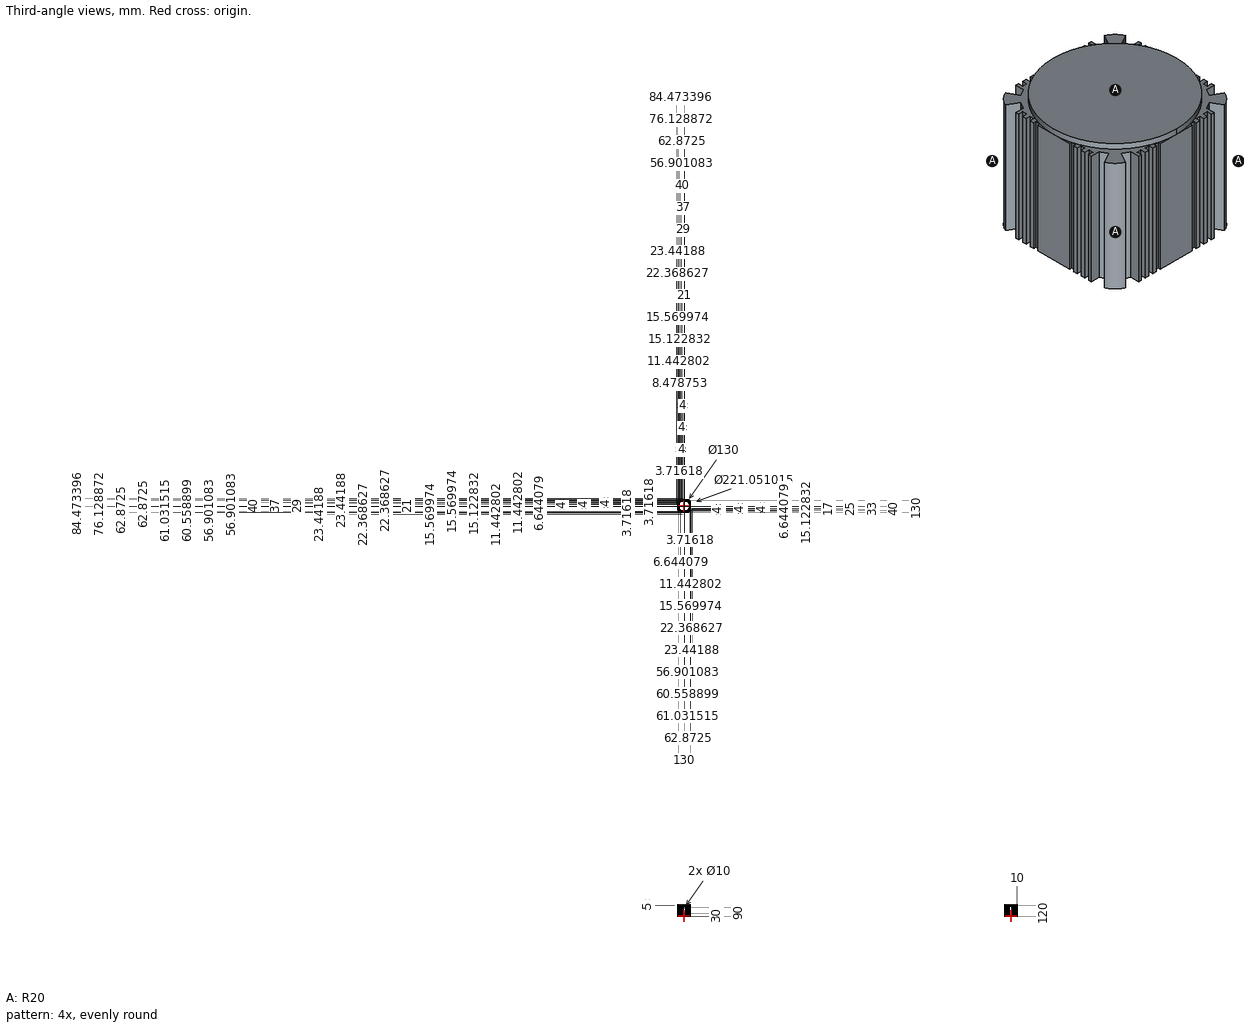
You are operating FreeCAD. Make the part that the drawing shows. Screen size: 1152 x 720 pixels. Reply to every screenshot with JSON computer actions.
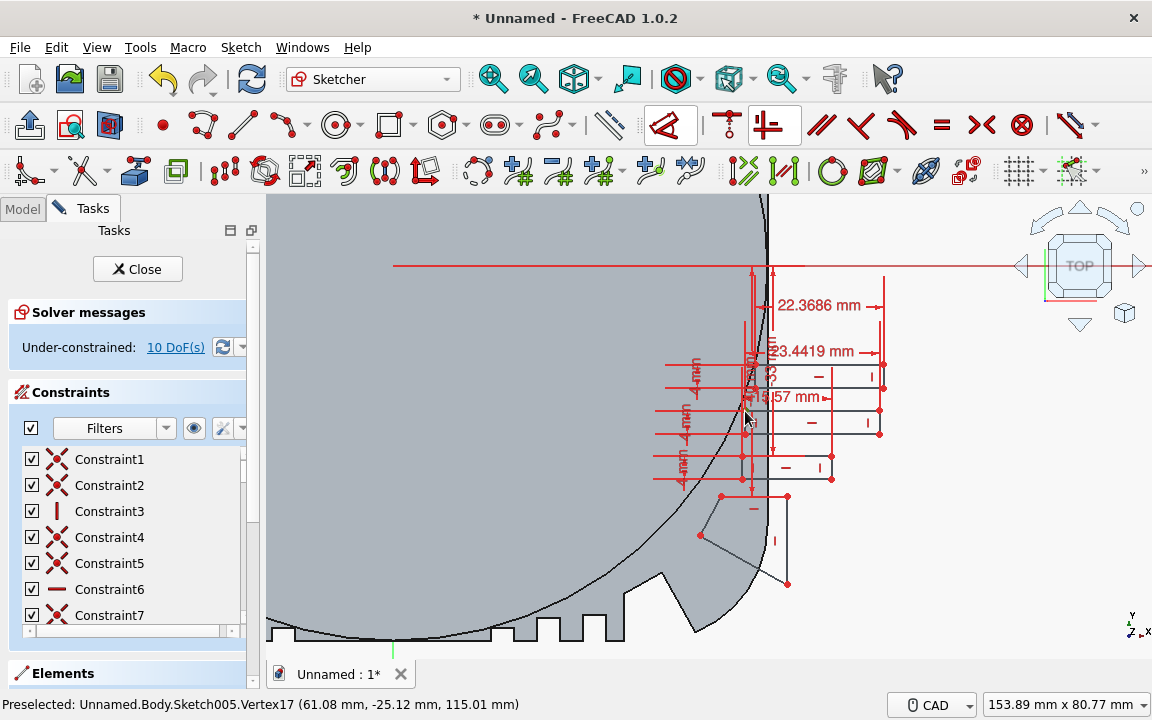
{"action": "left_click", "coordinate": [692, 126]}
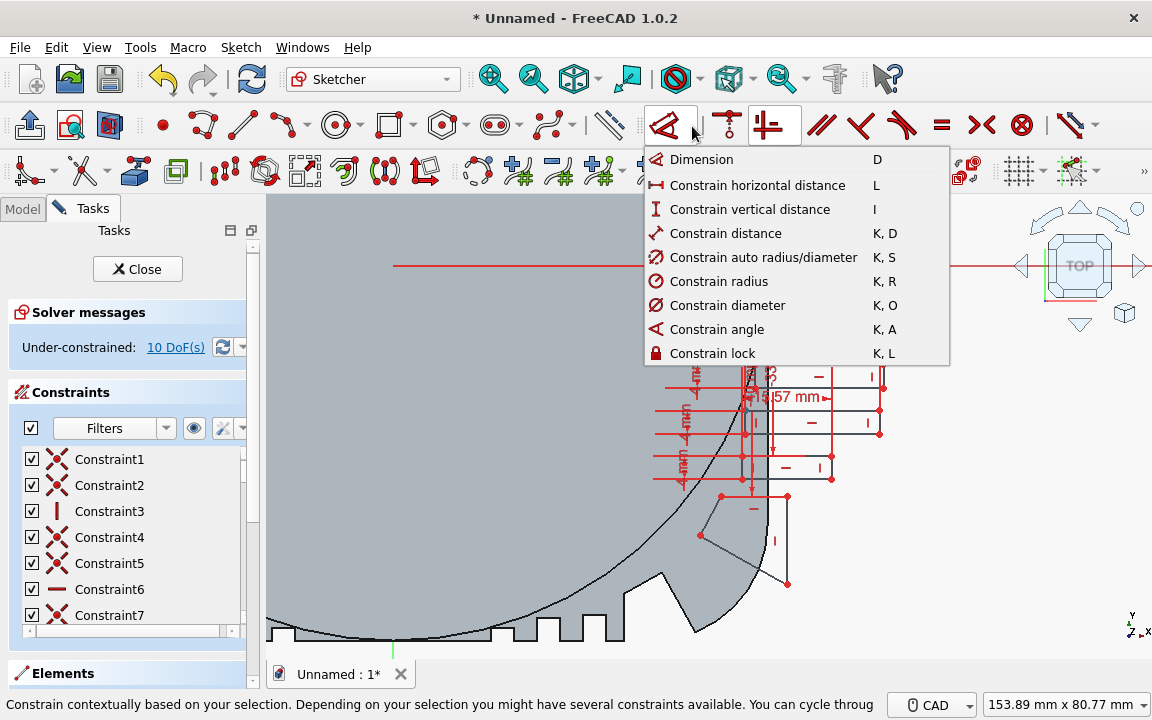
{"action": "left_click", "coordinate": [797, 209]}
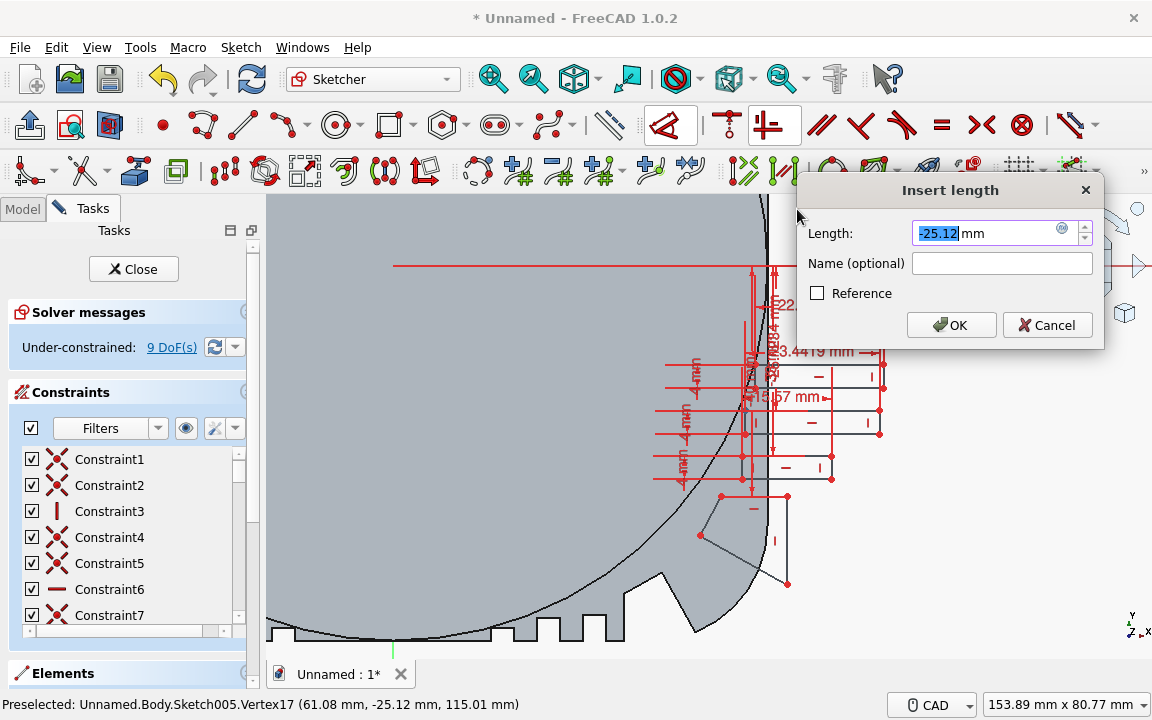
{"action": "type", "text": "-25"}
{"action": "key", "text": "Return"}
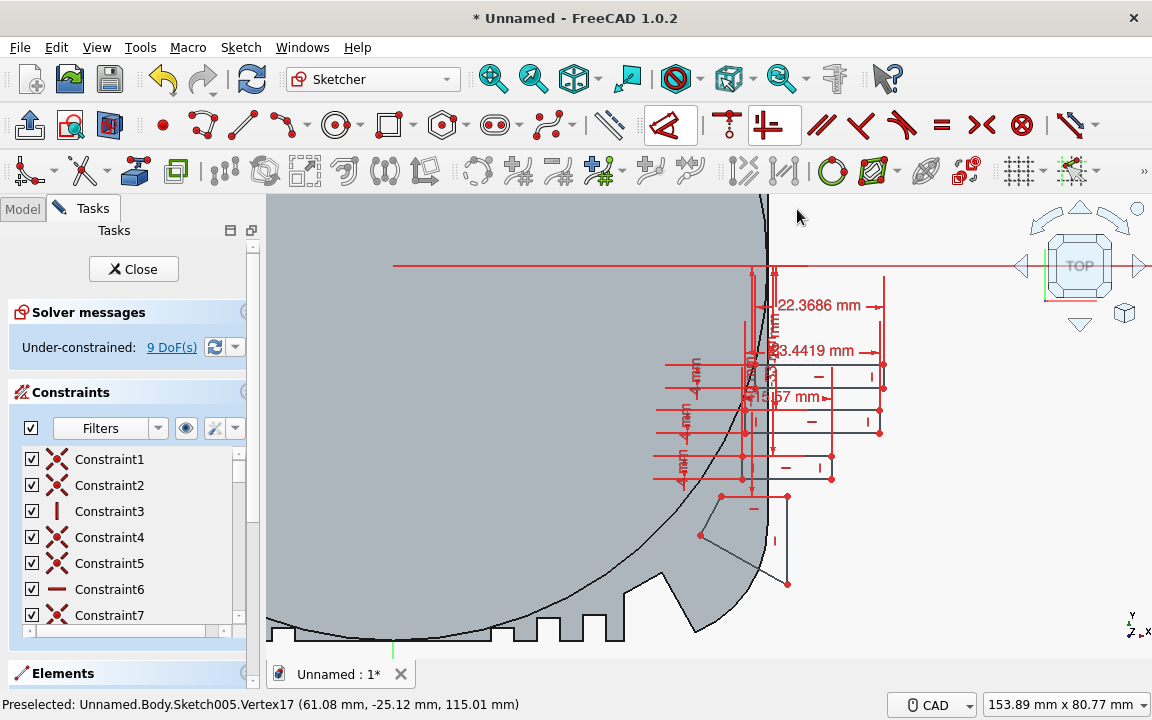
{"action": "left_click", "coordinate": [755, 365]}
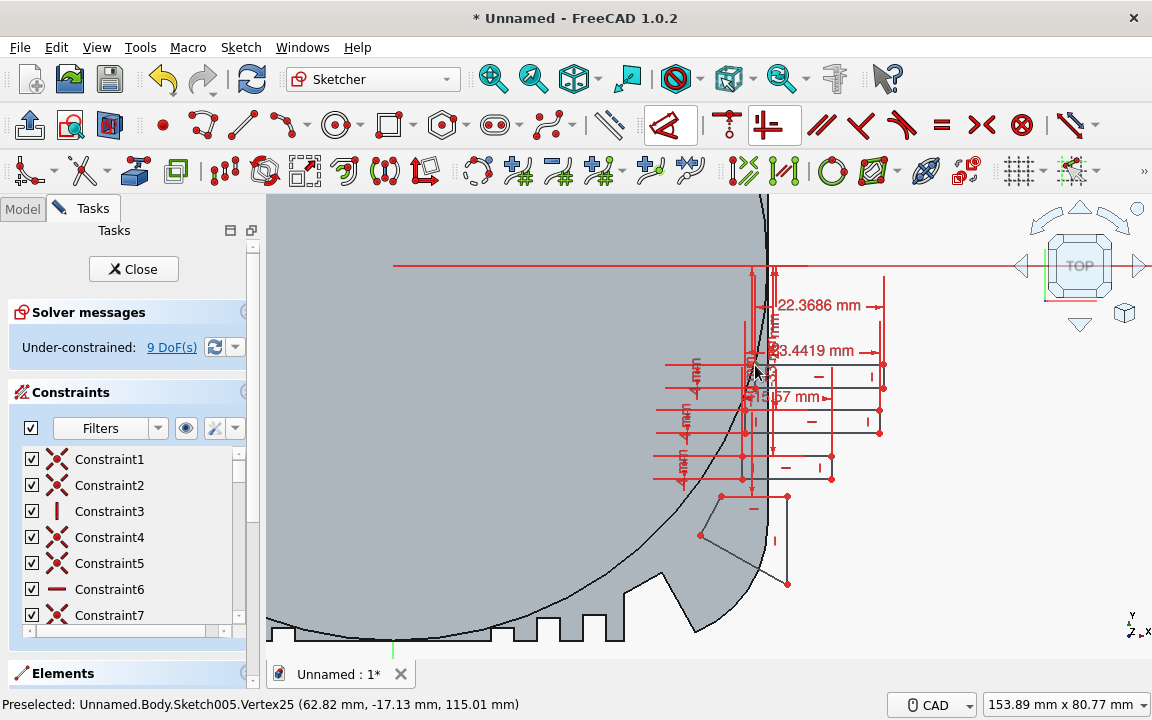
{"action": "left_click", "coordinate": [692, 126]}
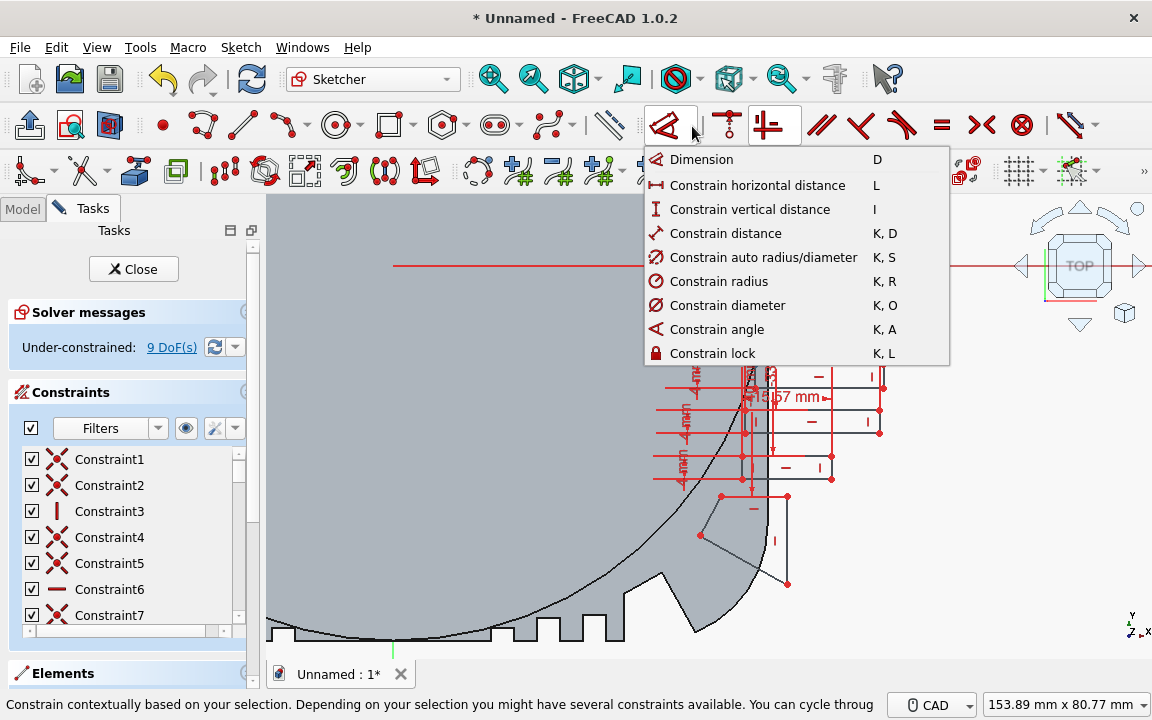
{"action": "left_click", "coordinate": [797, 209]}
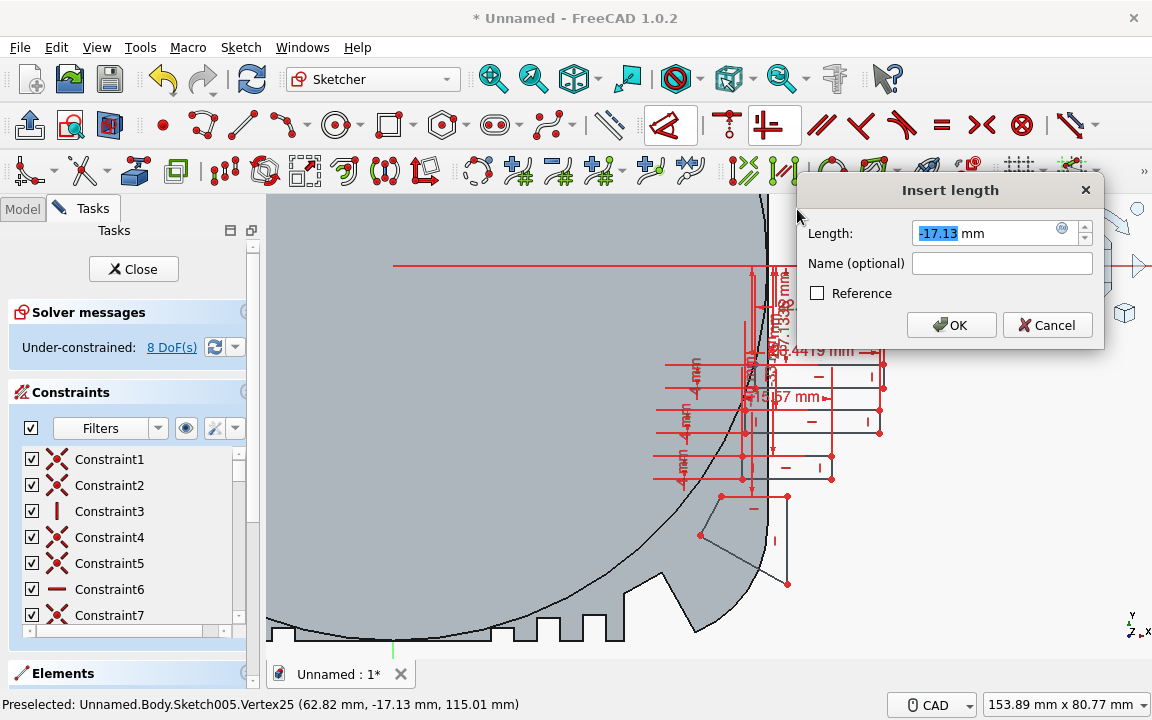
{"action": "type", "text": "-17"}
{"action": "key", "text": "Return"}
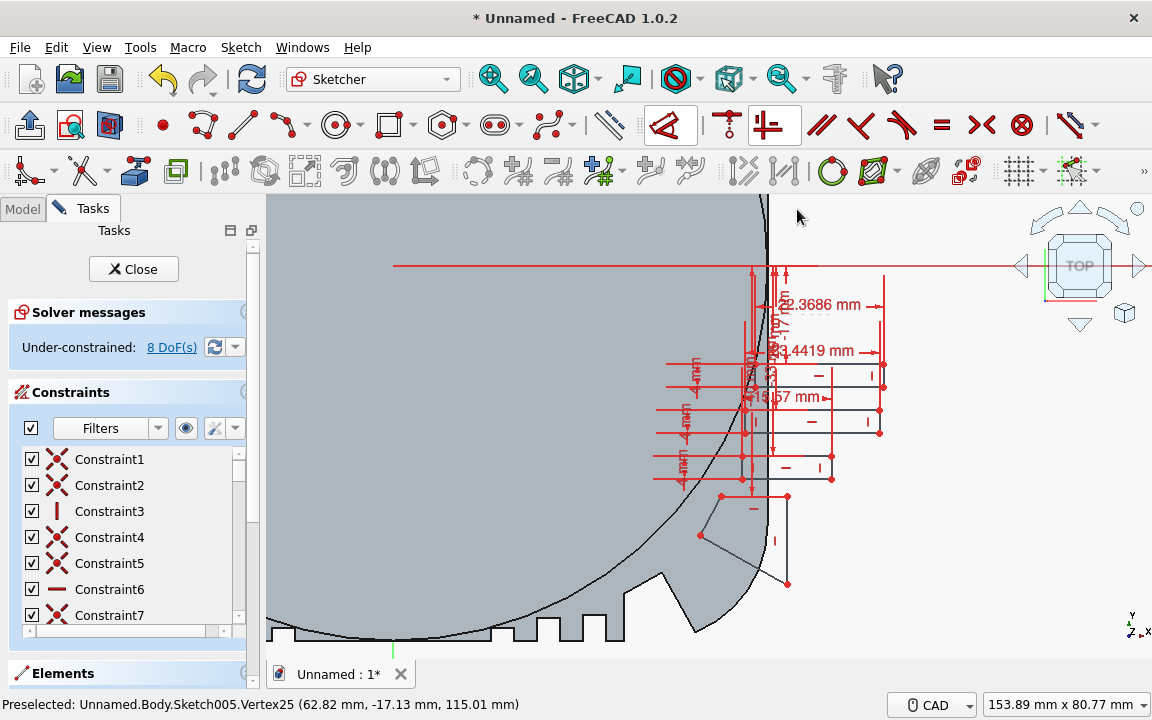
{"action": "left_click", "coordinate": [755, 364]}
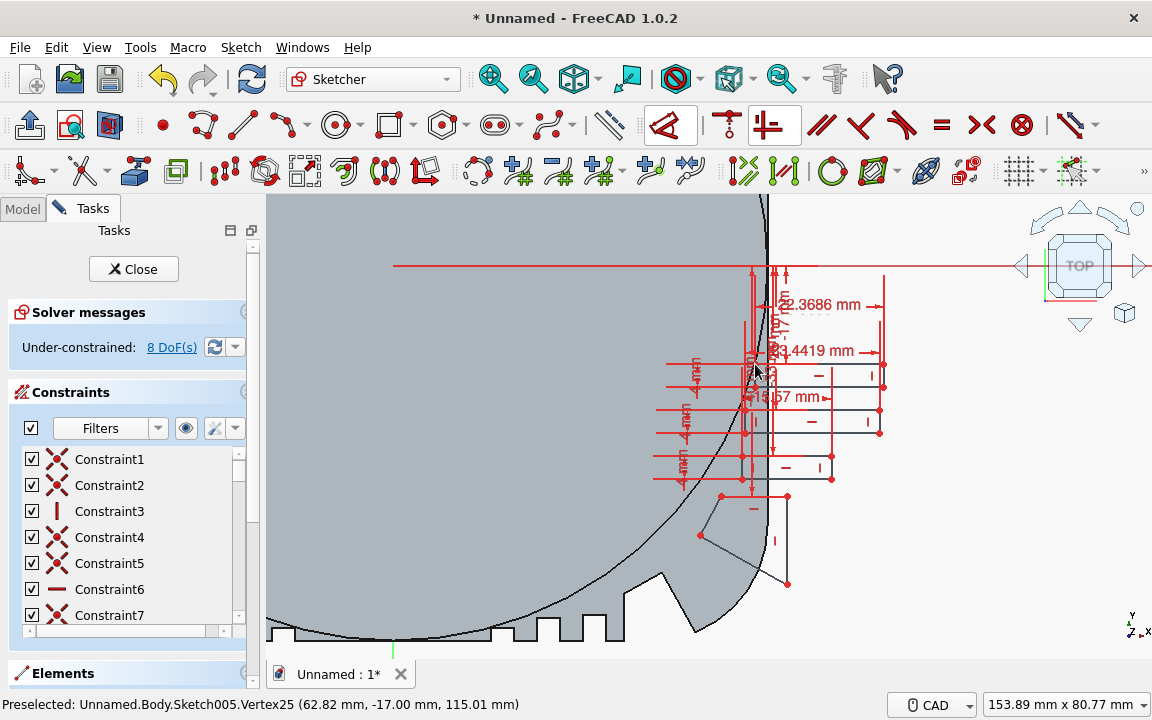
{"action": "key", "text": "l"}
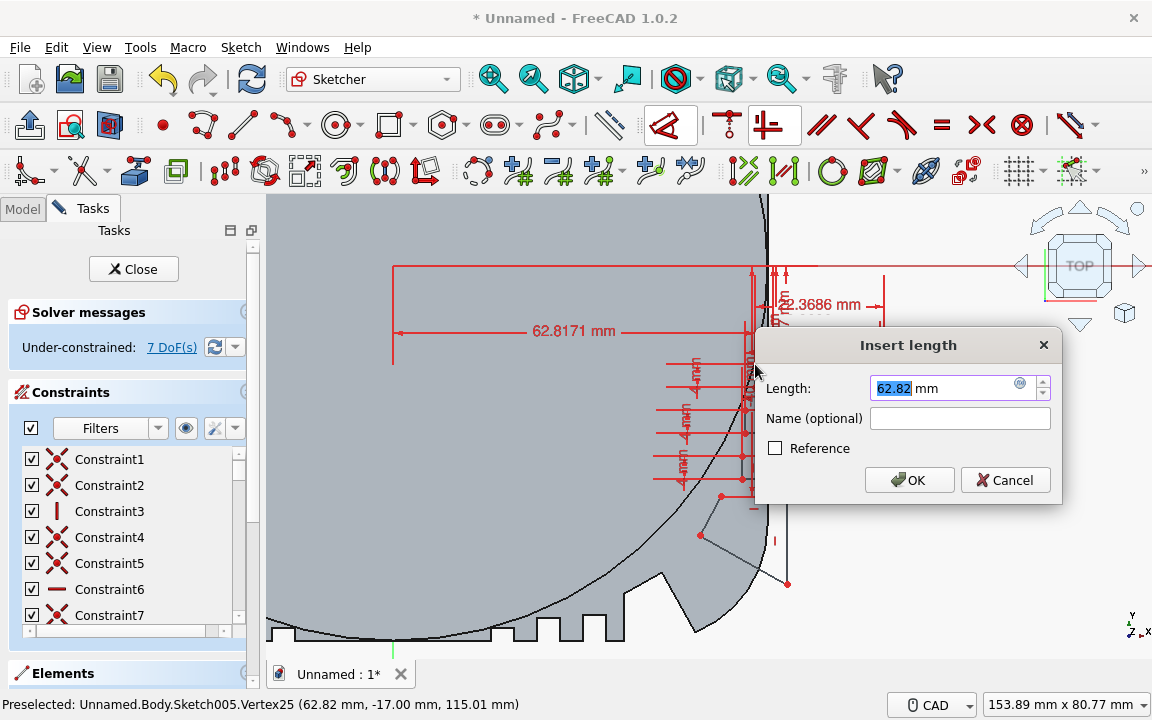
{"action": "type", "text": "62.8725"}
{"action": "key", "text": "Return"}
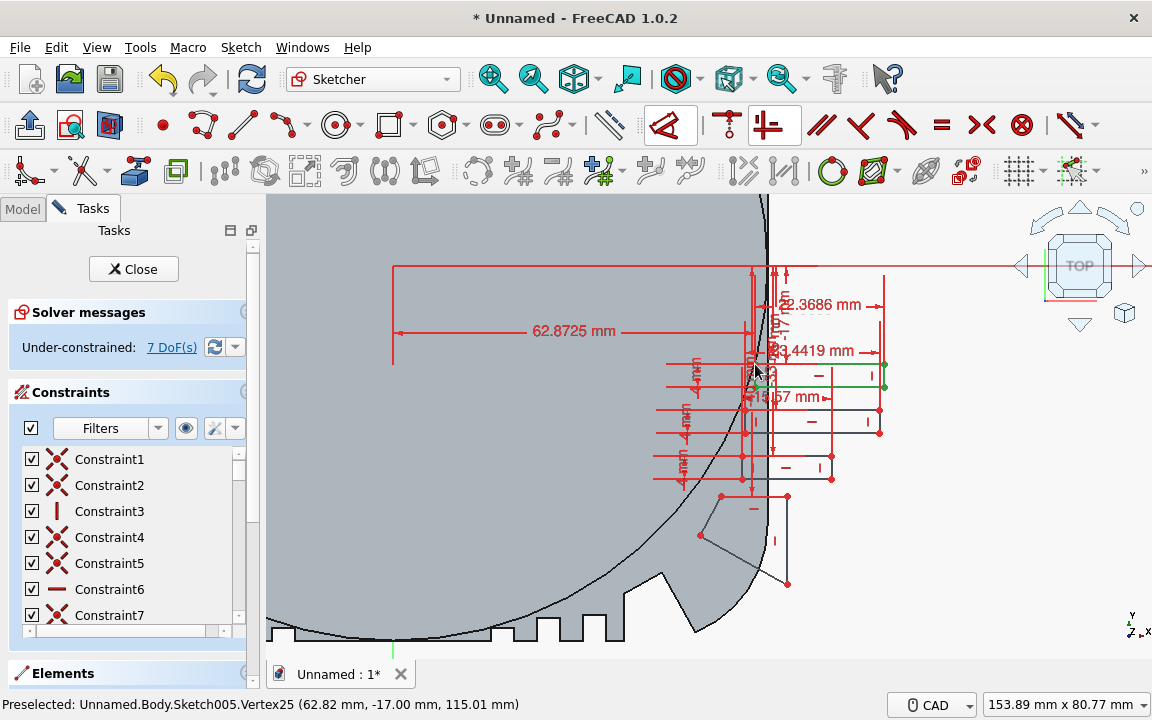
{"action": "scroll", "coordinate": [715, 508], "scroll_direction": "up", "scroll_amount": 4}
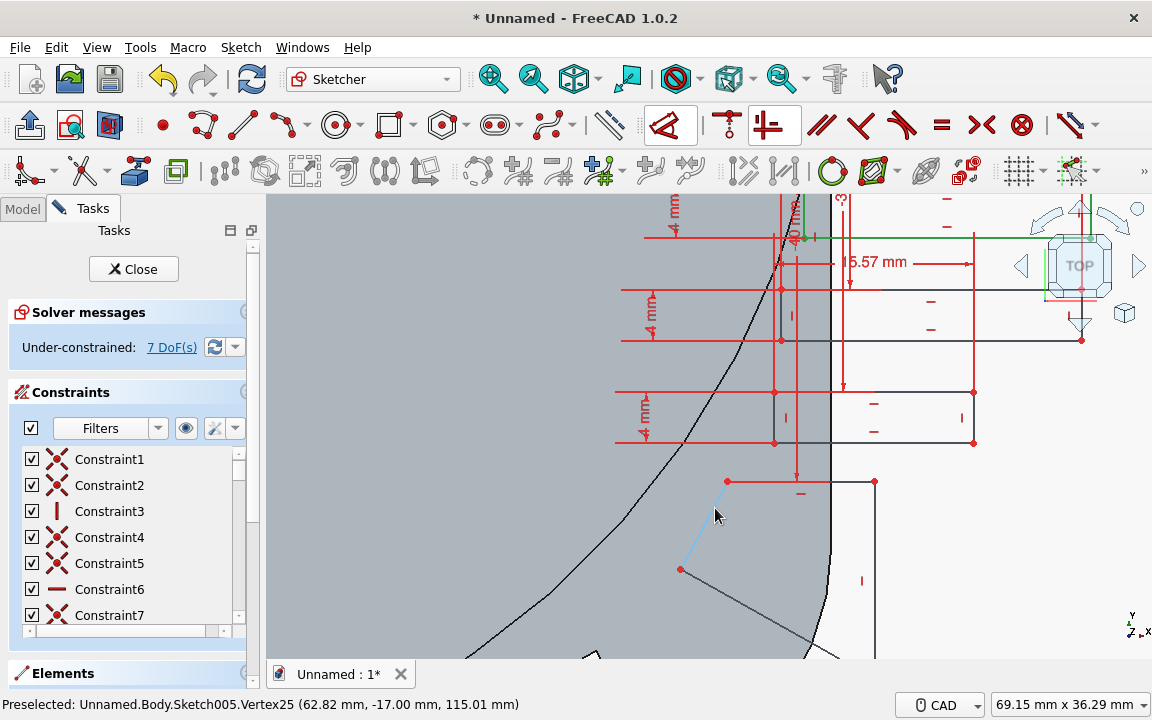
{"action": "left_click", "coordinate": [714, 508]}